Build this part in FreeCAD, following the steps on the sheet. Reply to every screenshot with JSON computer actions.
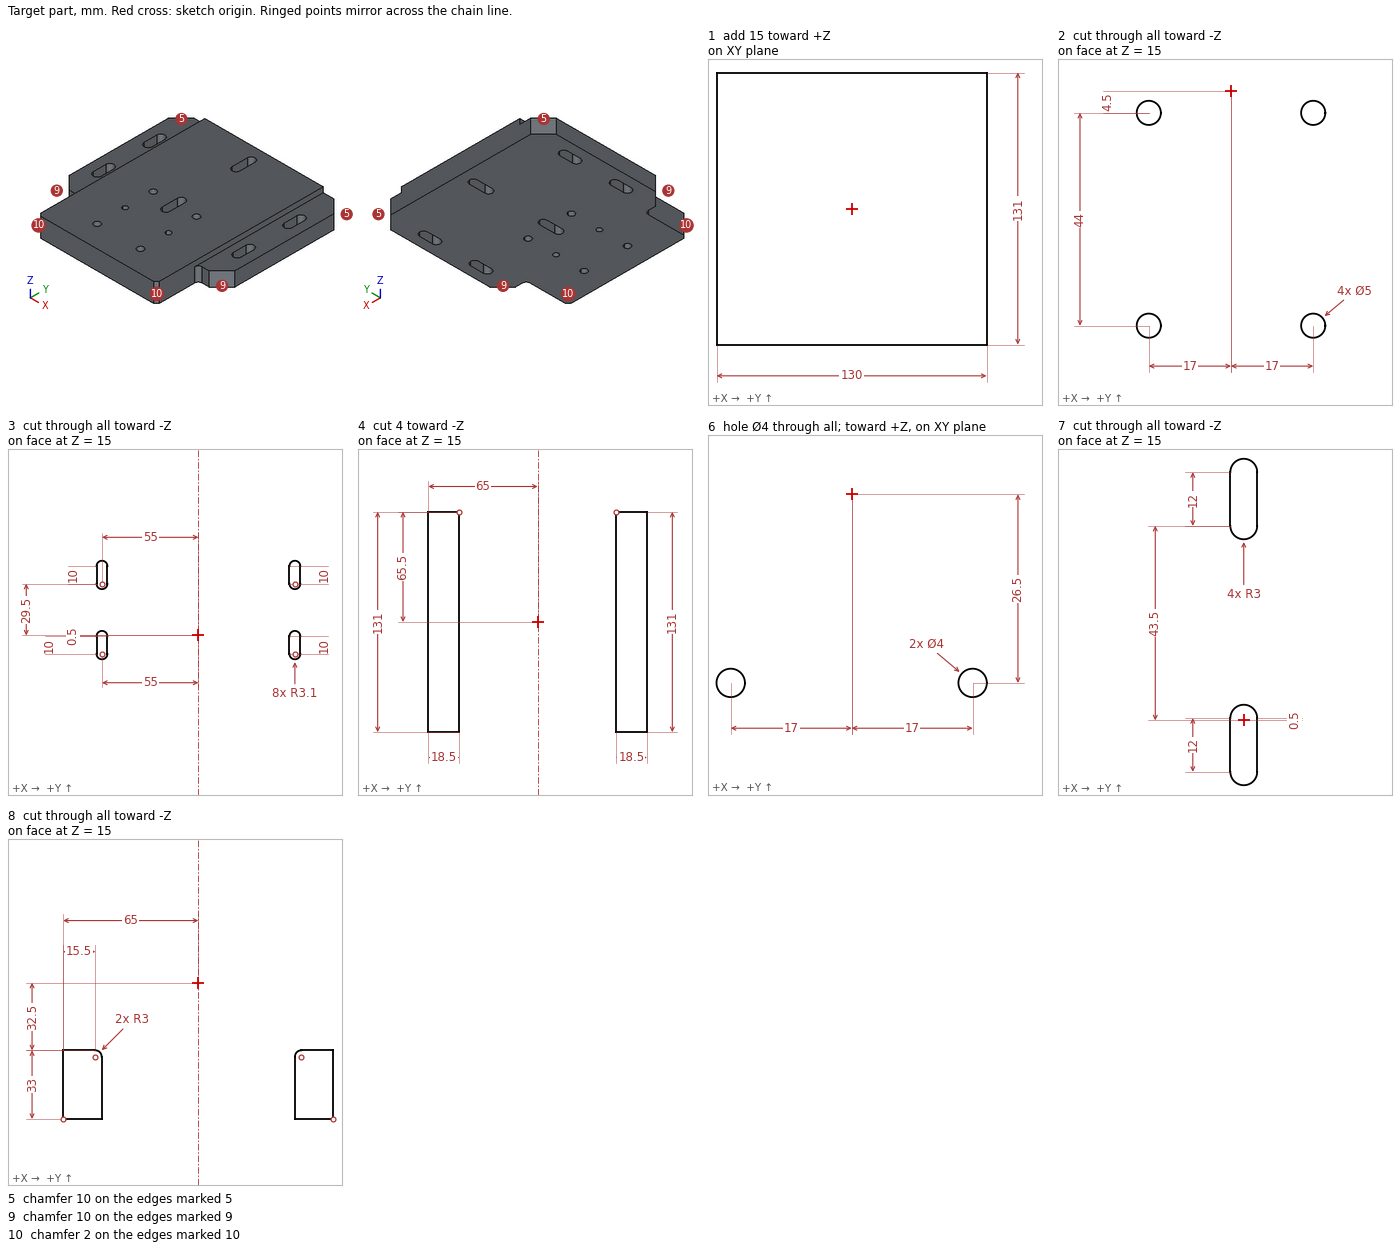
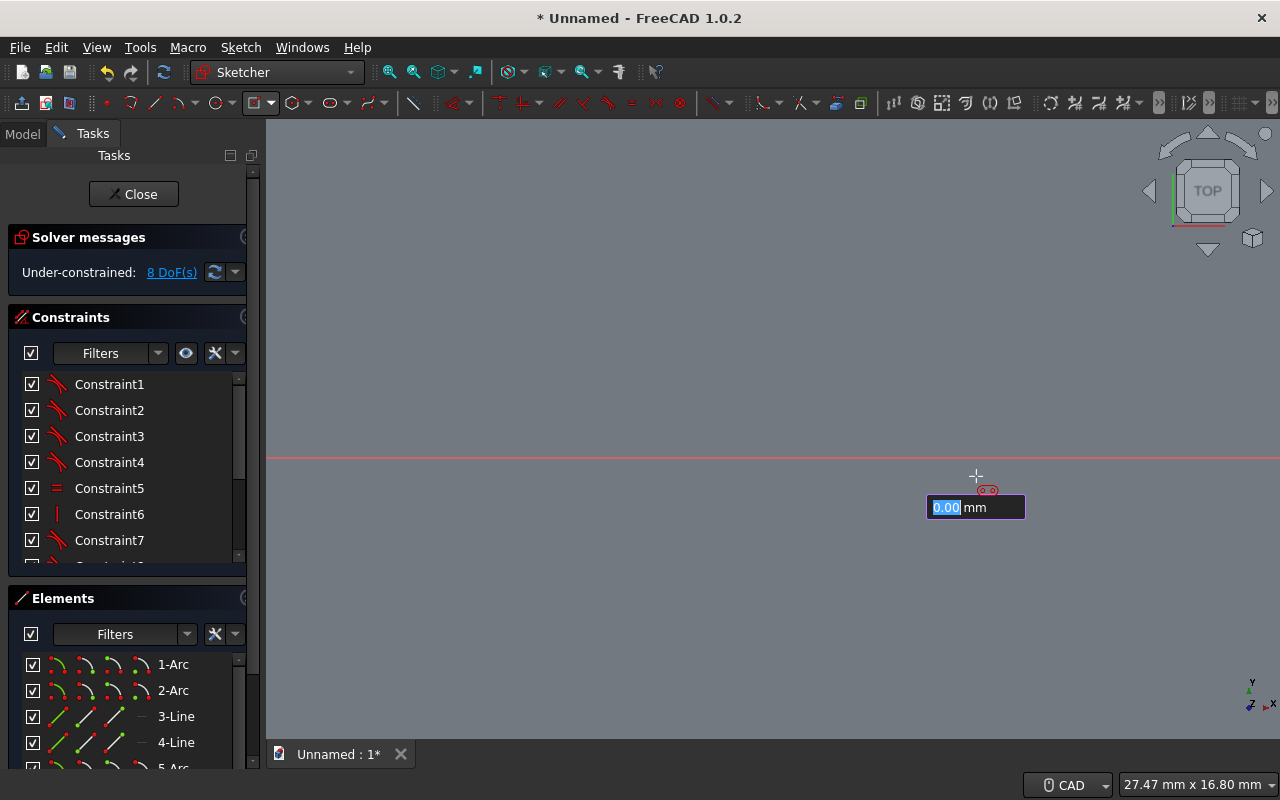
{"action": "scroll", "coordinate": [980, 508], "scroll_direction": "down", "scroll_amount": 10}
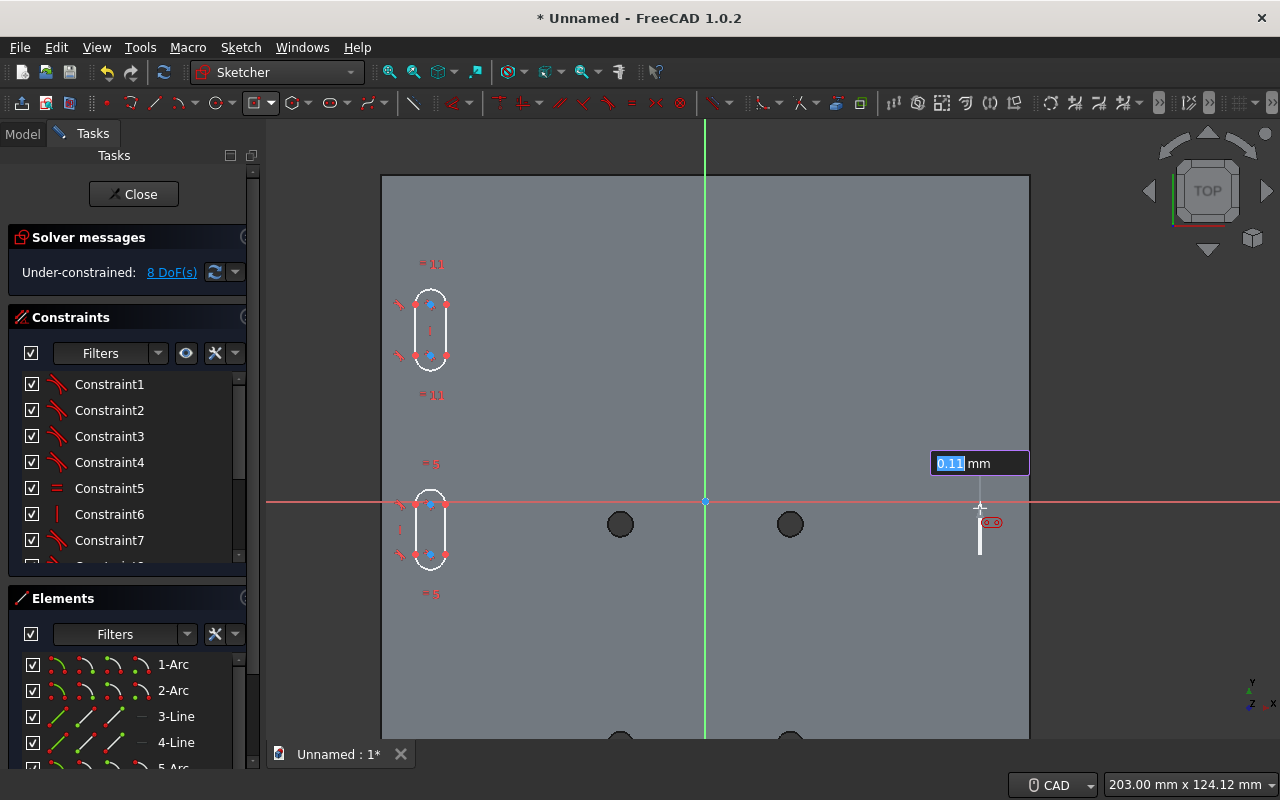
{"action": "left_click", "coordinate": [965, 529]}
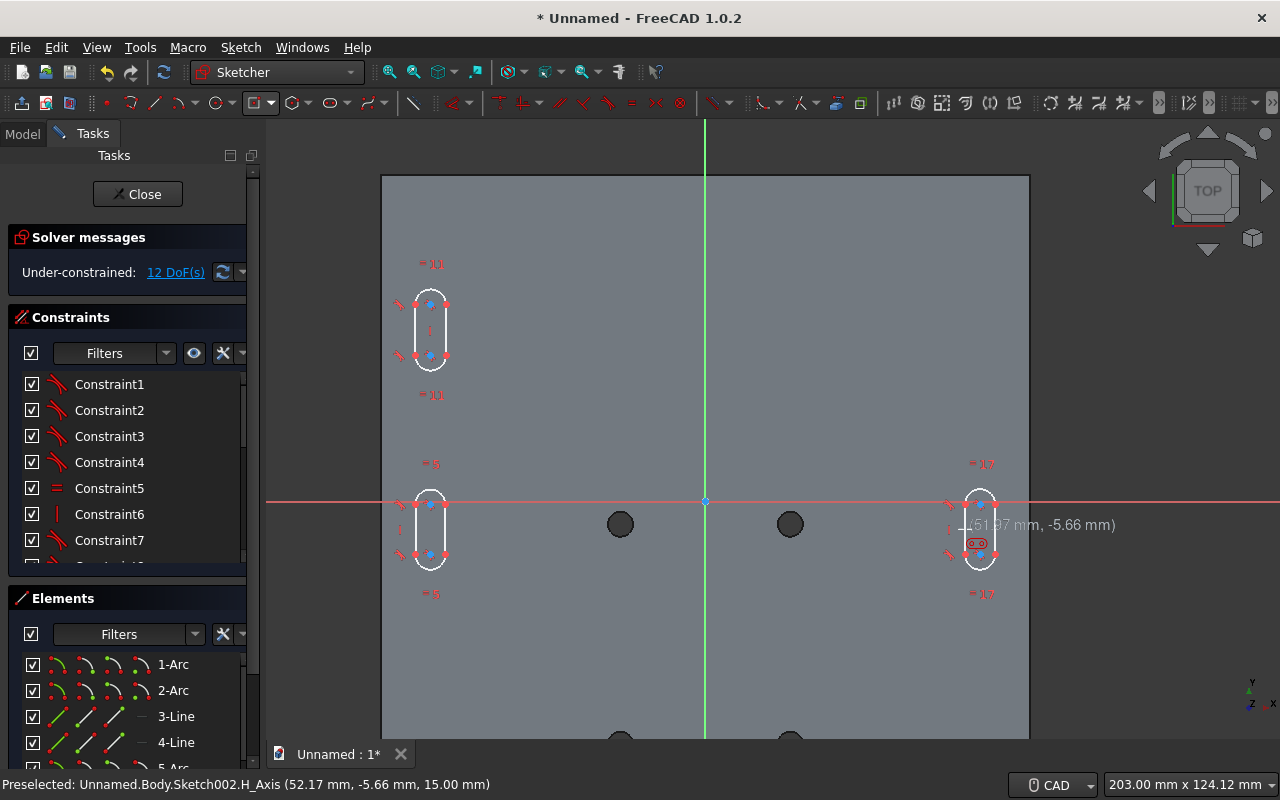
{"action": "scroll", "coordinate": [980, 354], "scroll_direction": "up", "scroll_amount": 2}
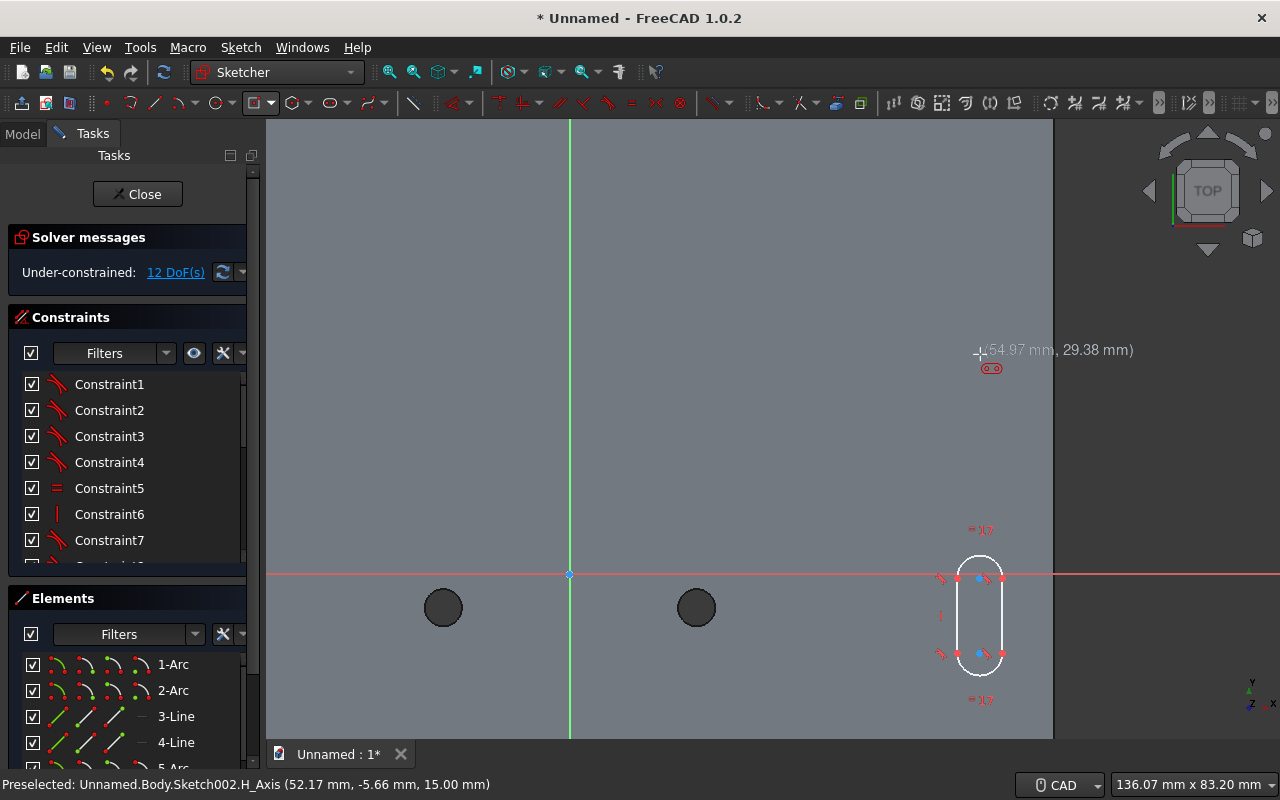
{"action": "left_click", "coordinate": [980, 354]}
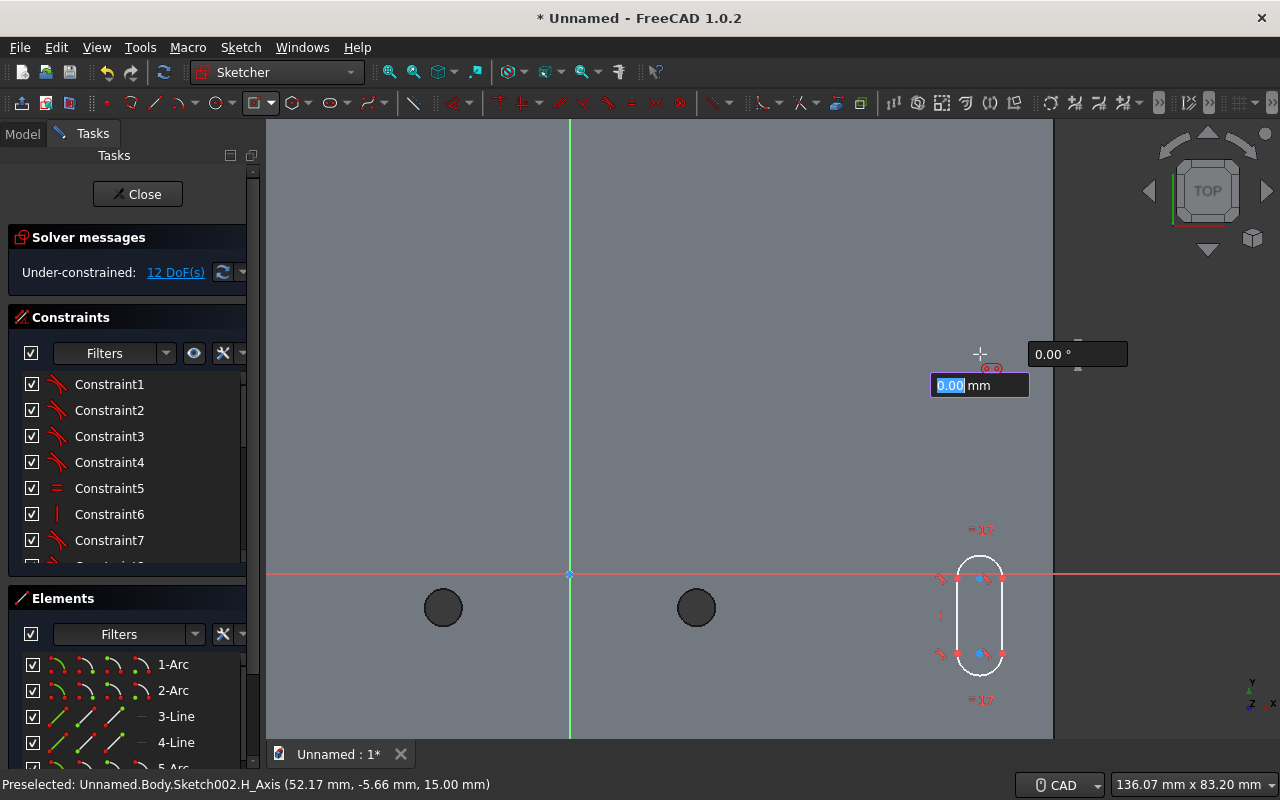
{"action": "left_click", "coordinate": [980, 280]}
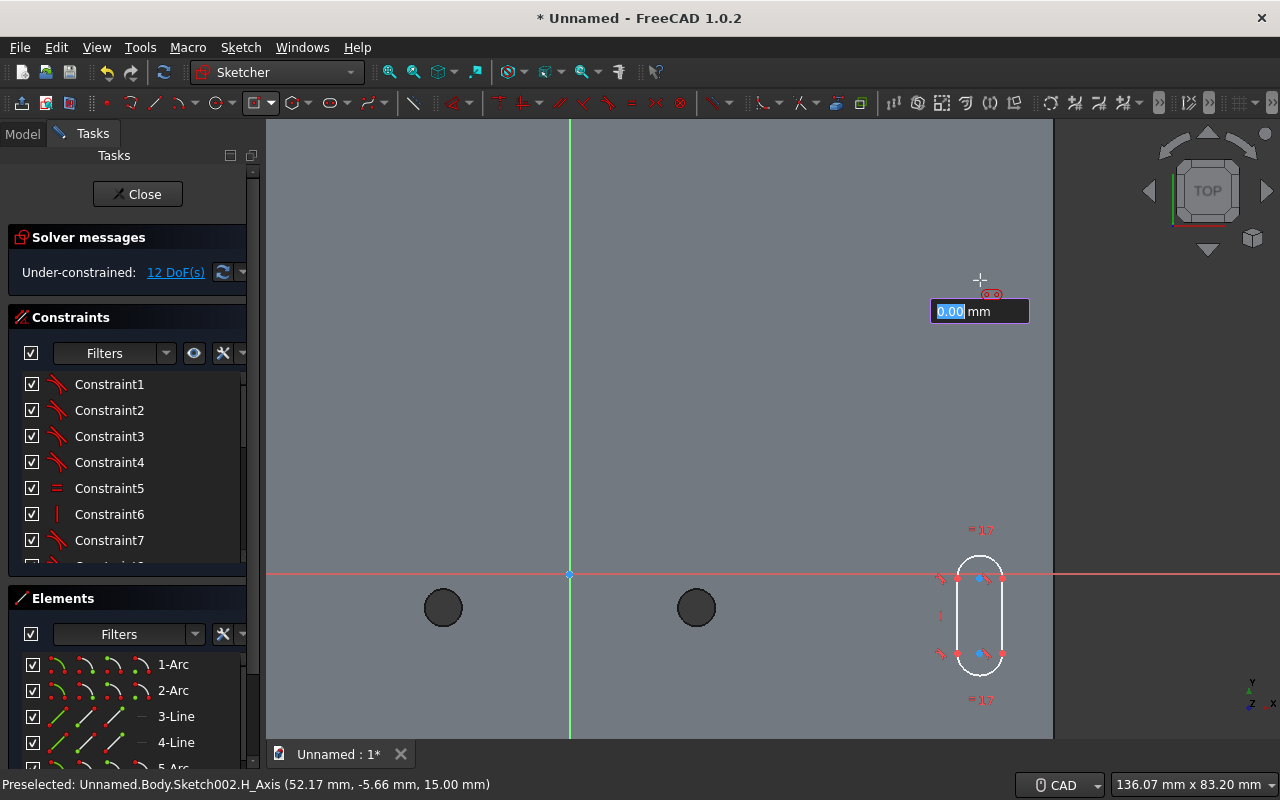
{"action": "left_click", "coordinate": [957, 317]}
{"action": "key", "text": "Escape"}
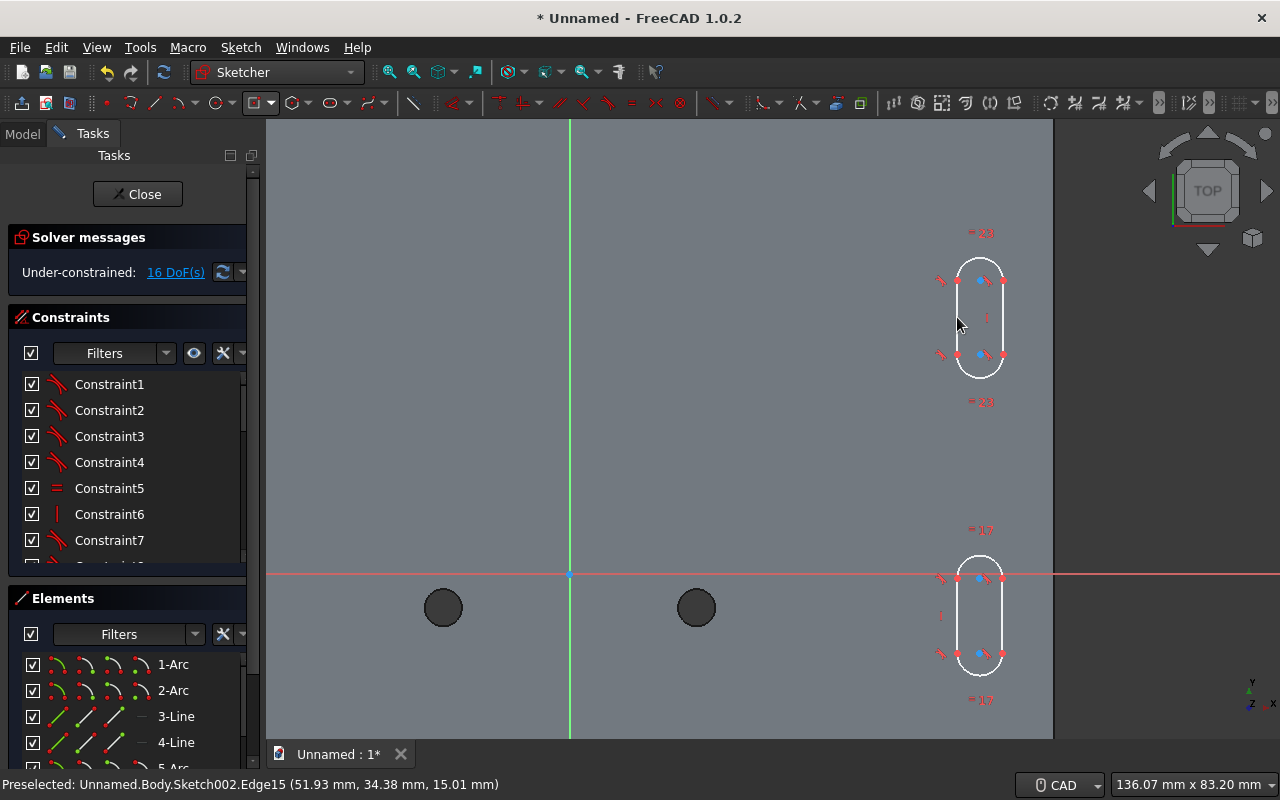
{"action": "scroll", "coordinate": [978, 353], "scroll_direction": "down", "scroll_amount": 2}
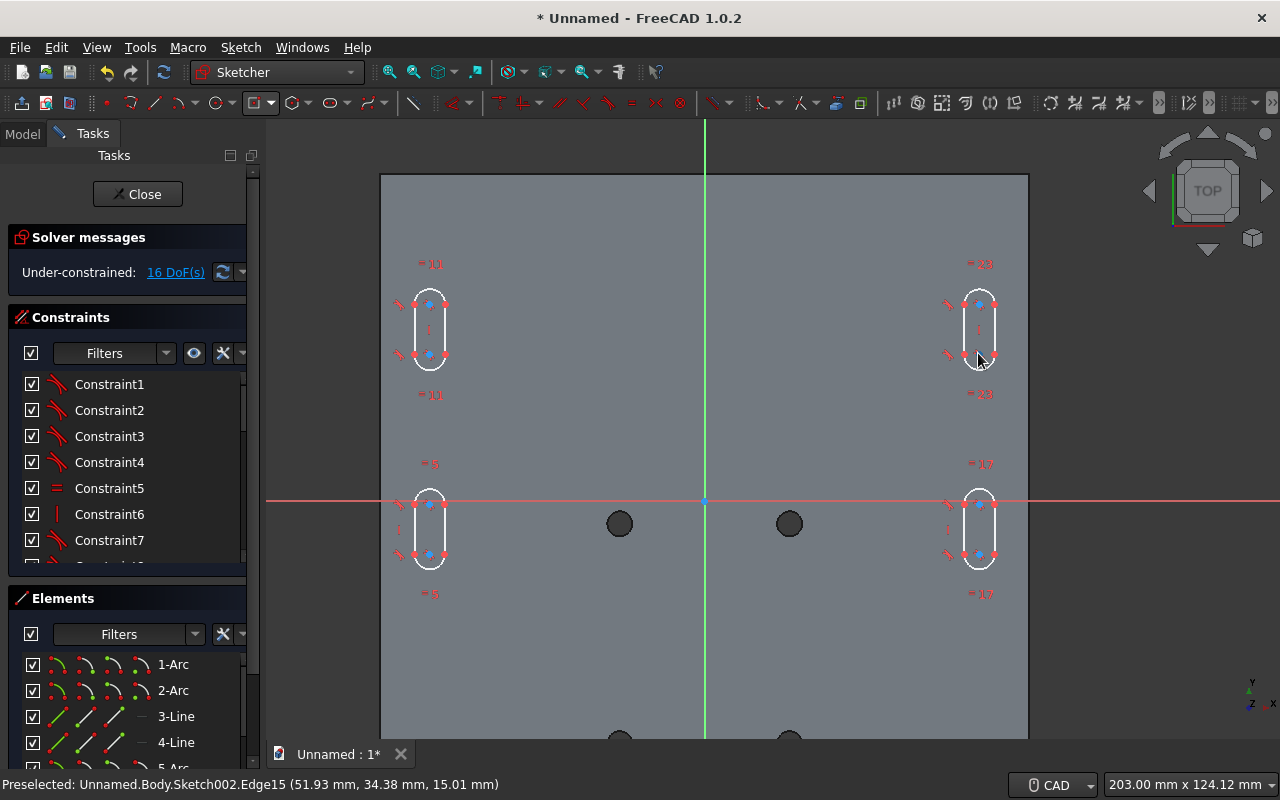
{"action": "left_click", "coordinate": [421, 567]}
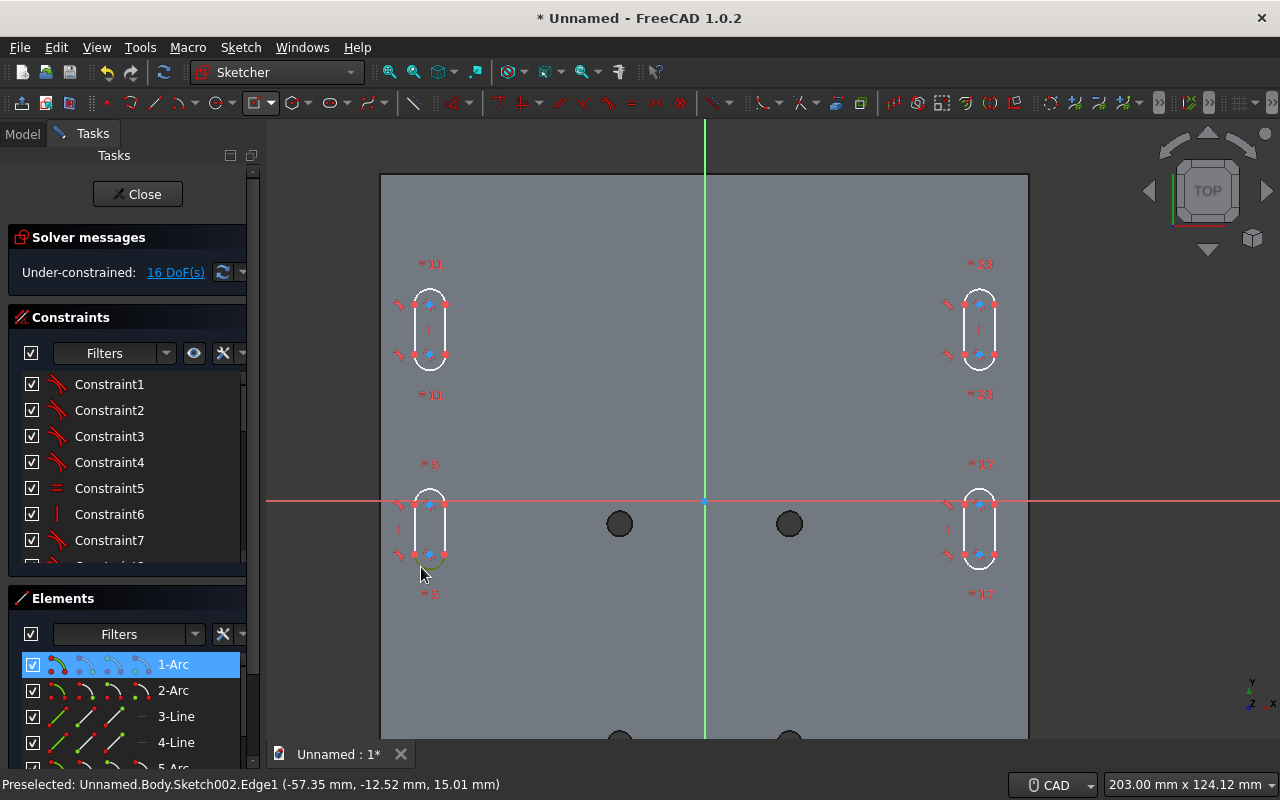
{"action": "left_click", "coordinate": [421, 367]}